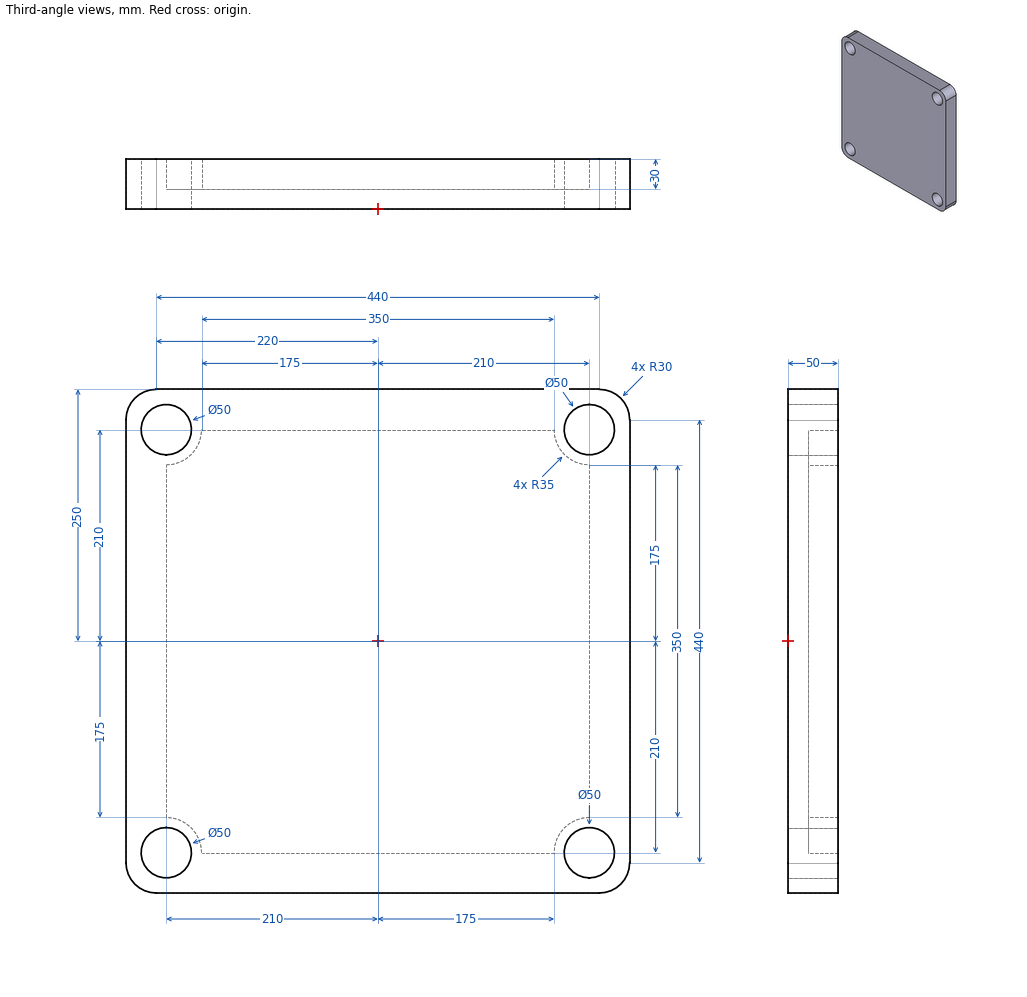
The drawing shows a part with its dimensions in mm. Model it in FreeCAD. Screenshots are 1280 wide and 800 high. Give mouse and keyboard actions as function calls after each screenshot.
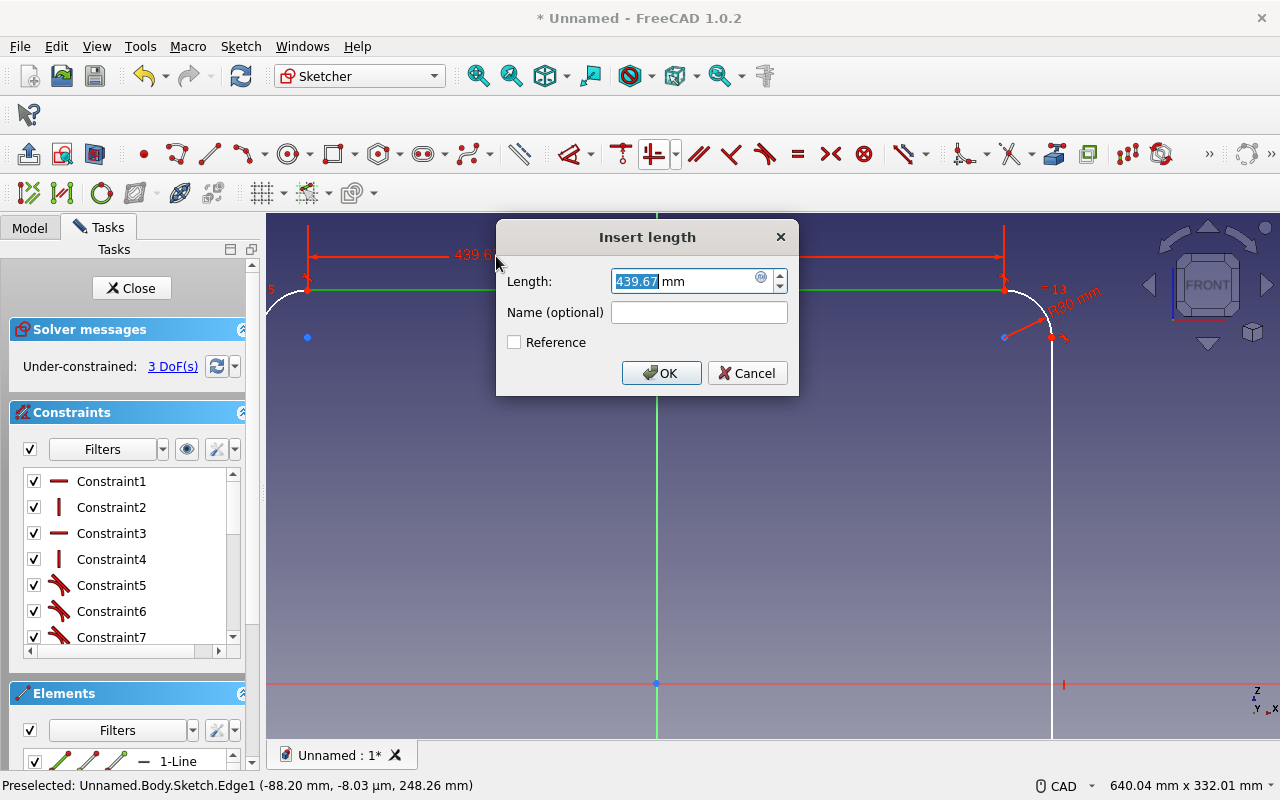
text(440)
key(Return)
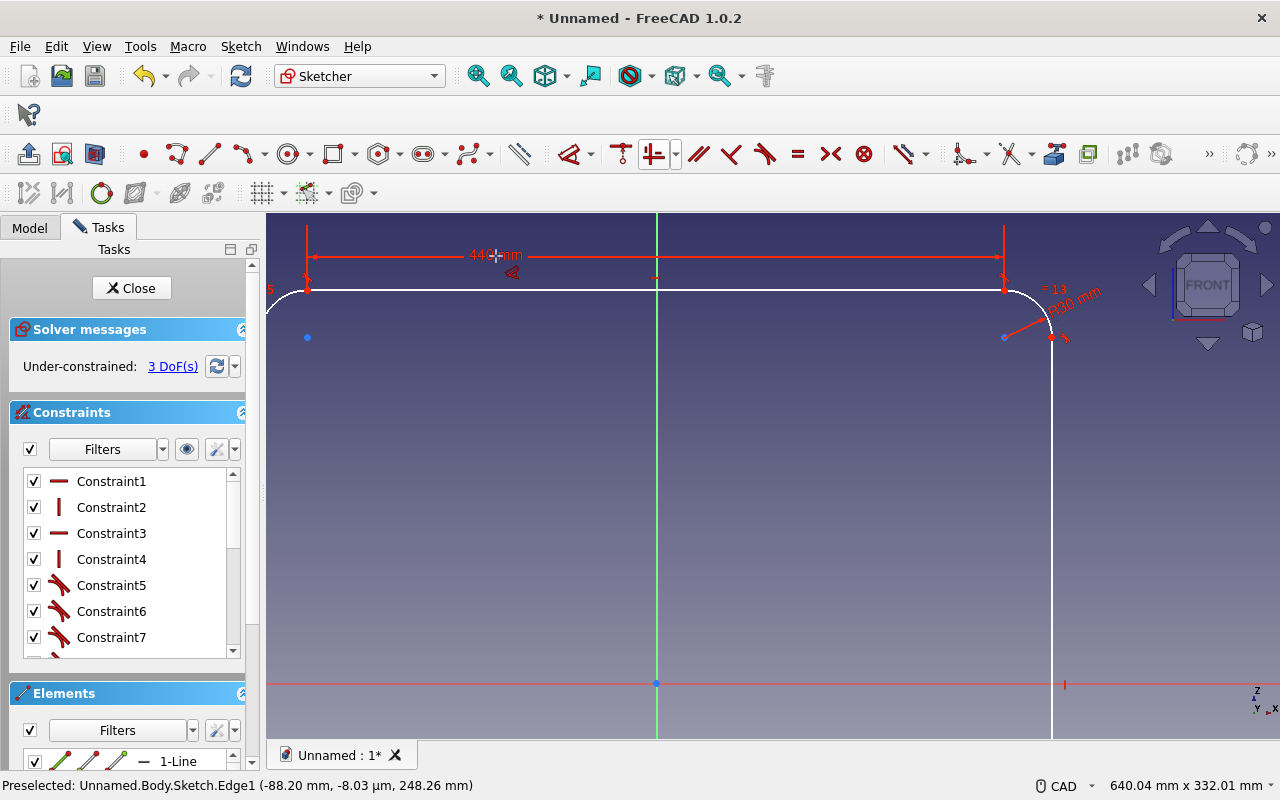
click(1052, 546)
click(1086, 524)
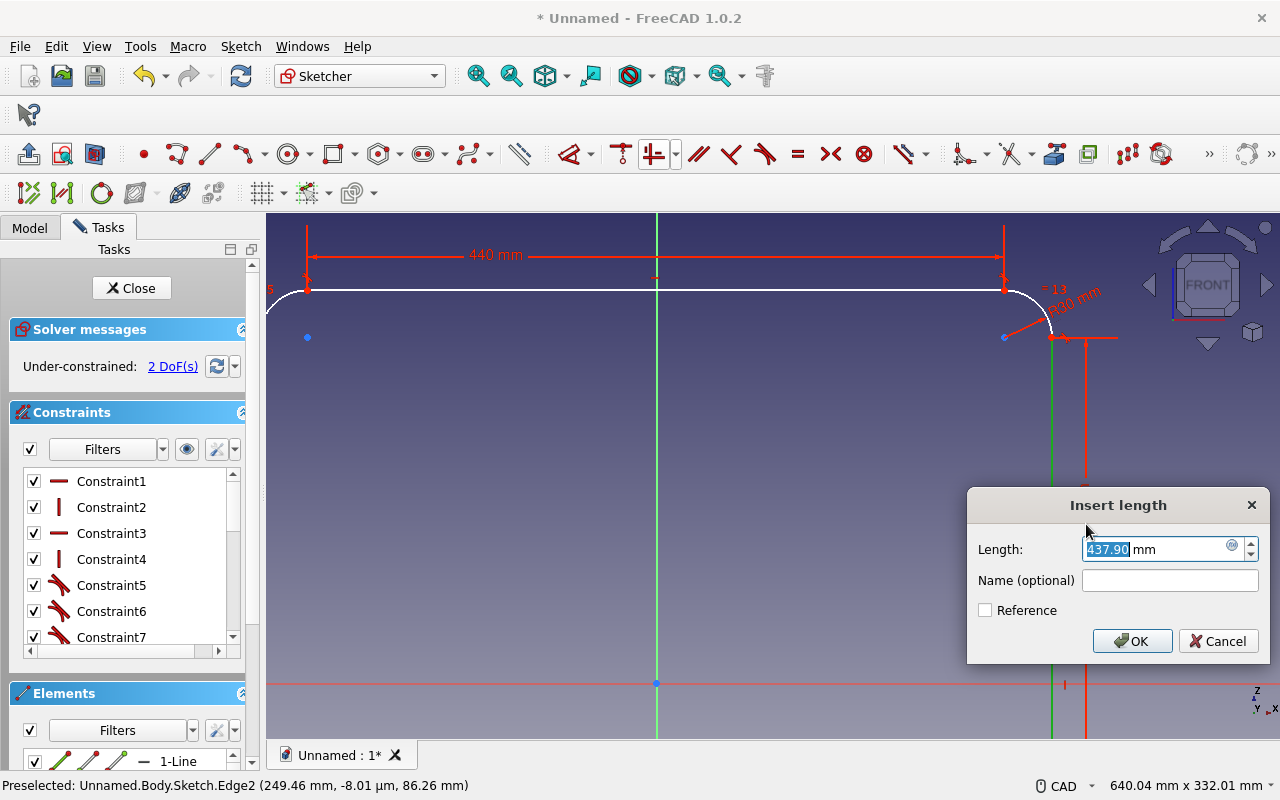
text(440)
key(Return)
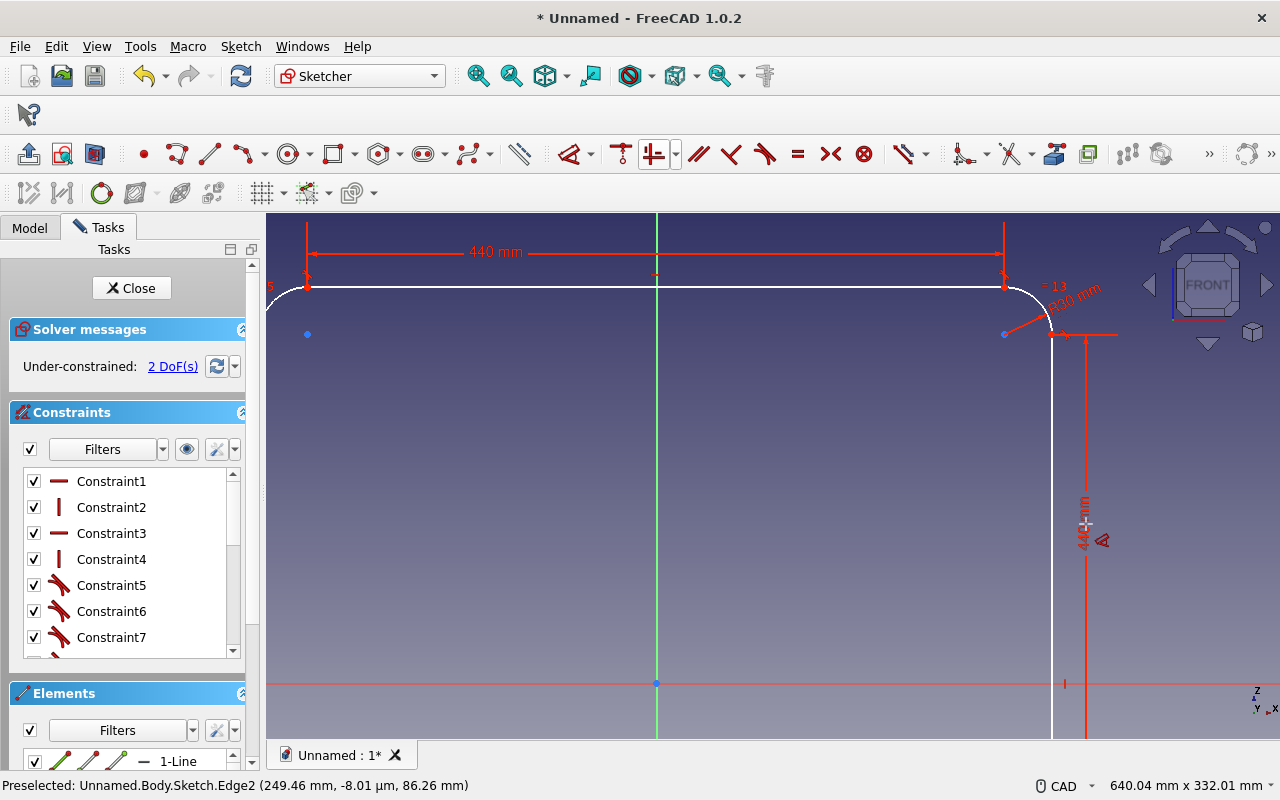
click(307, 287)
click(402, 253)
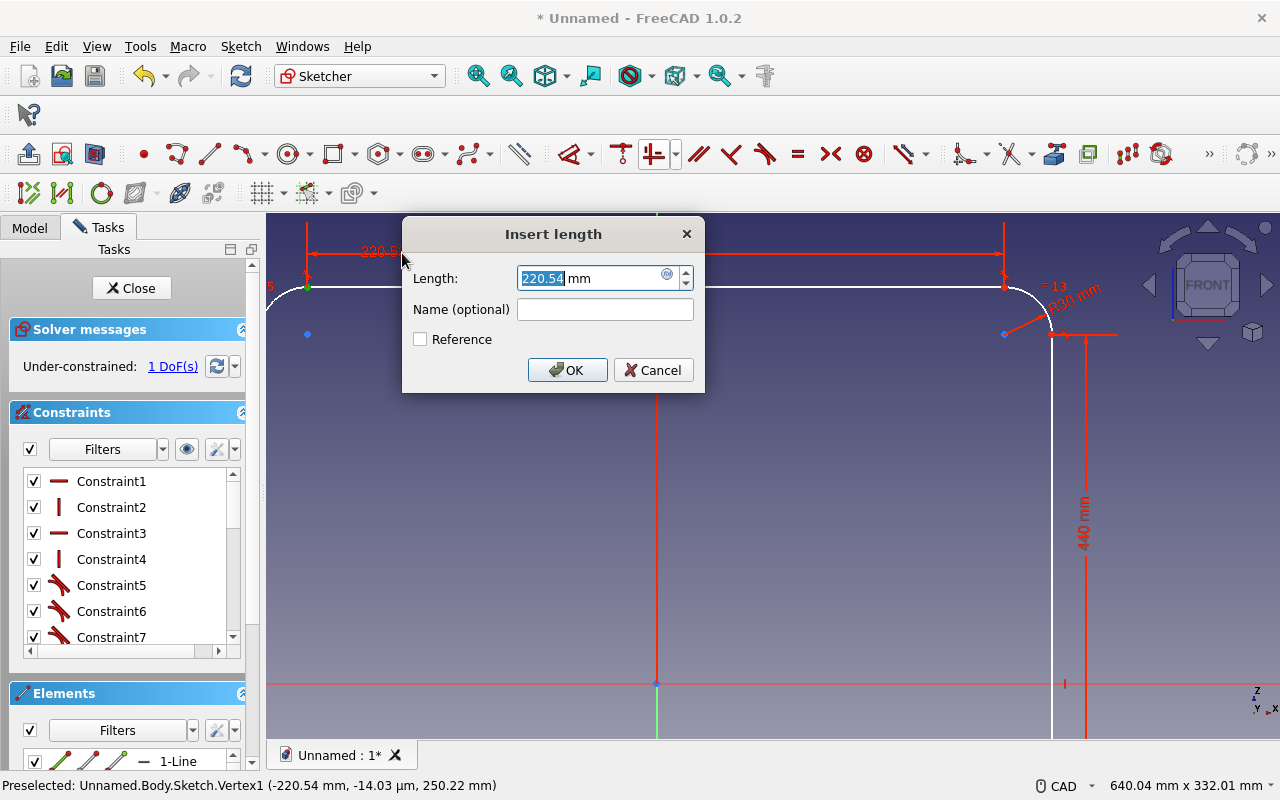
text(220)
key(Return)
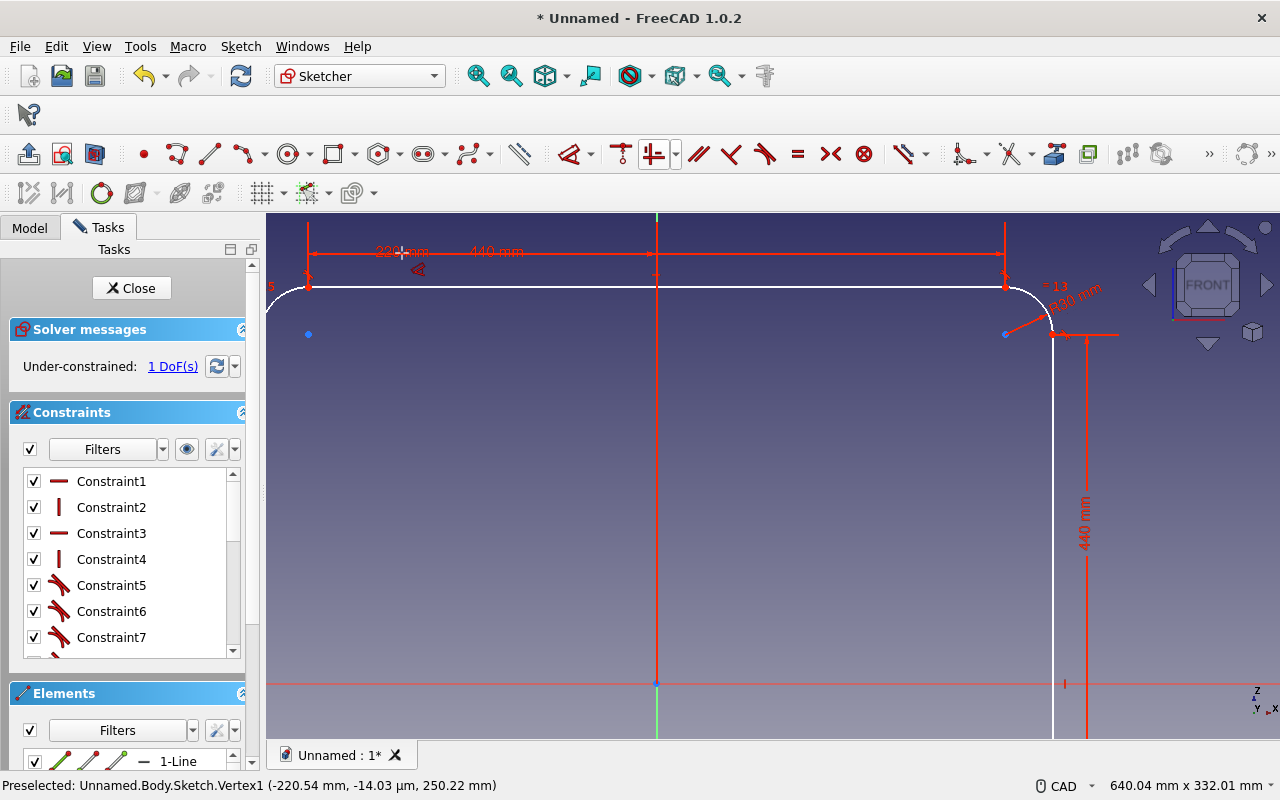
click(308, 287)
click(691, 485)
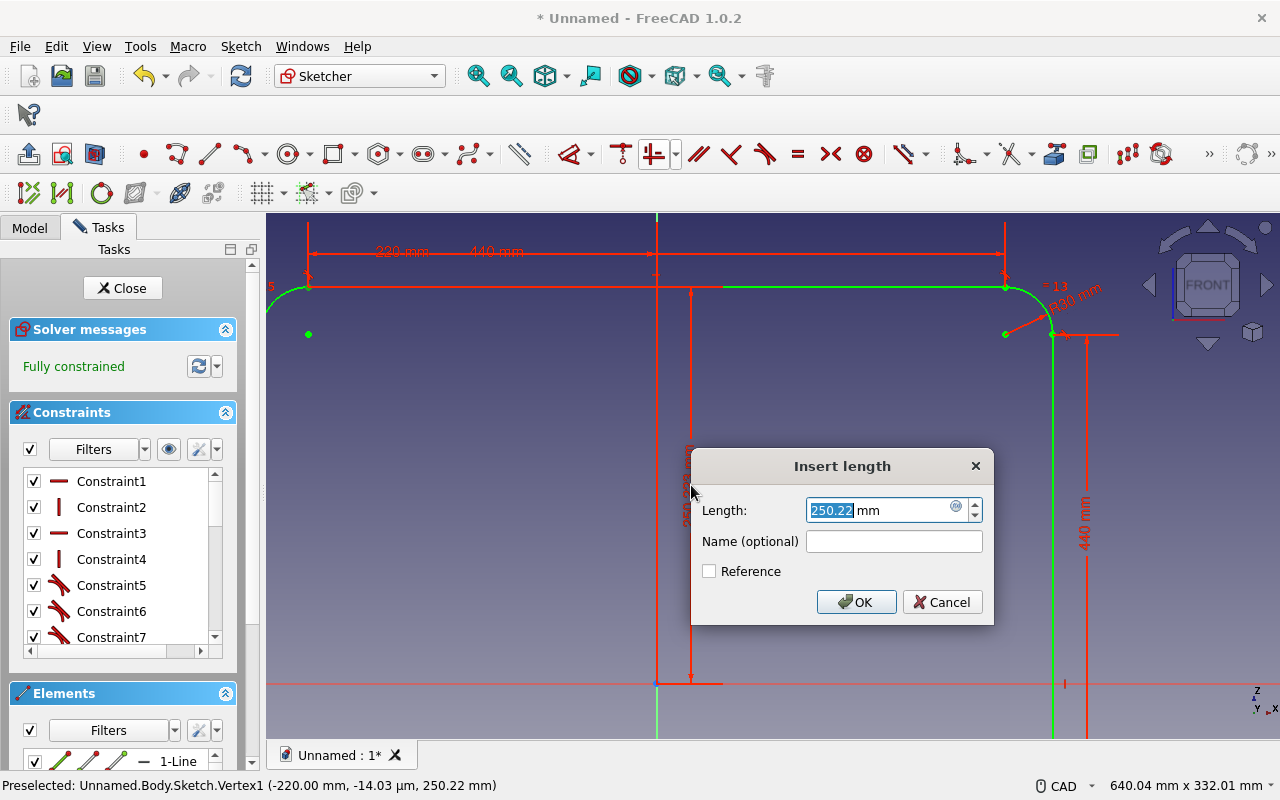
text(250)
key(Return)
key(Escape)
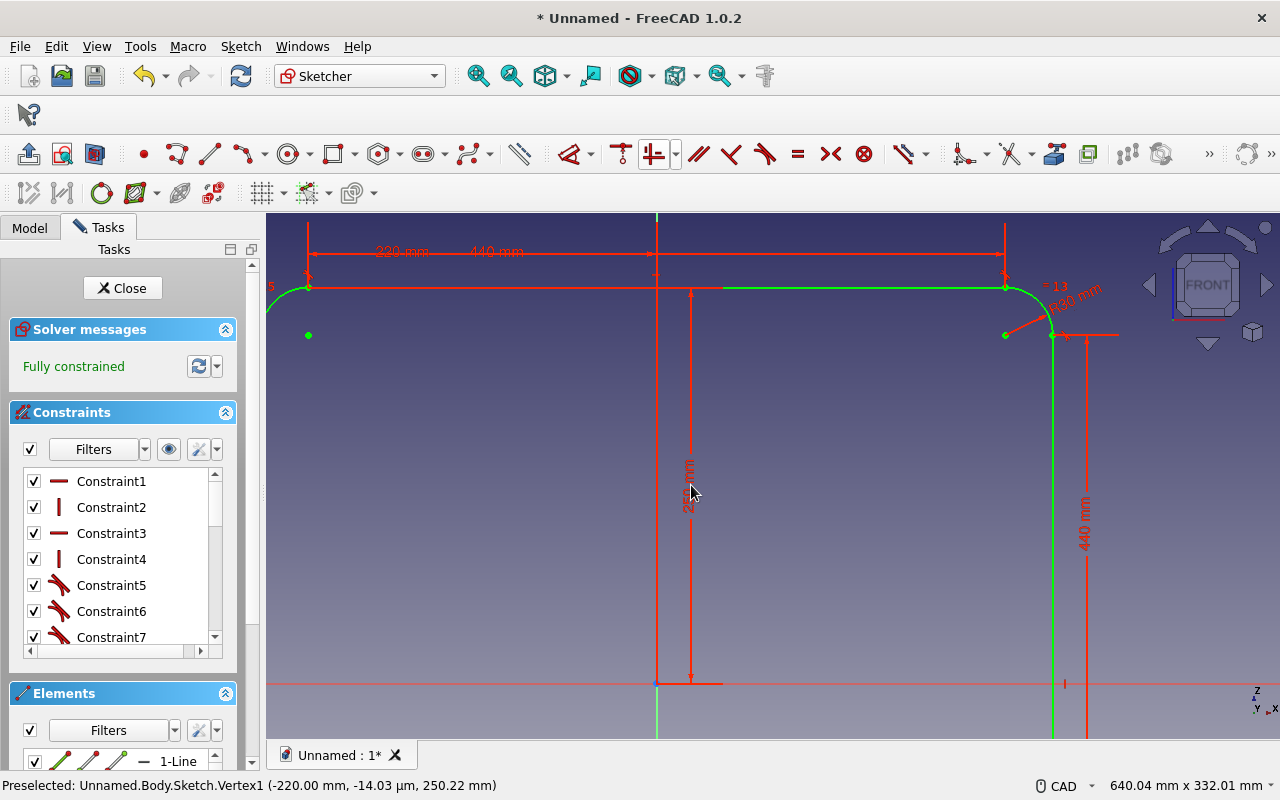
click(123, 288)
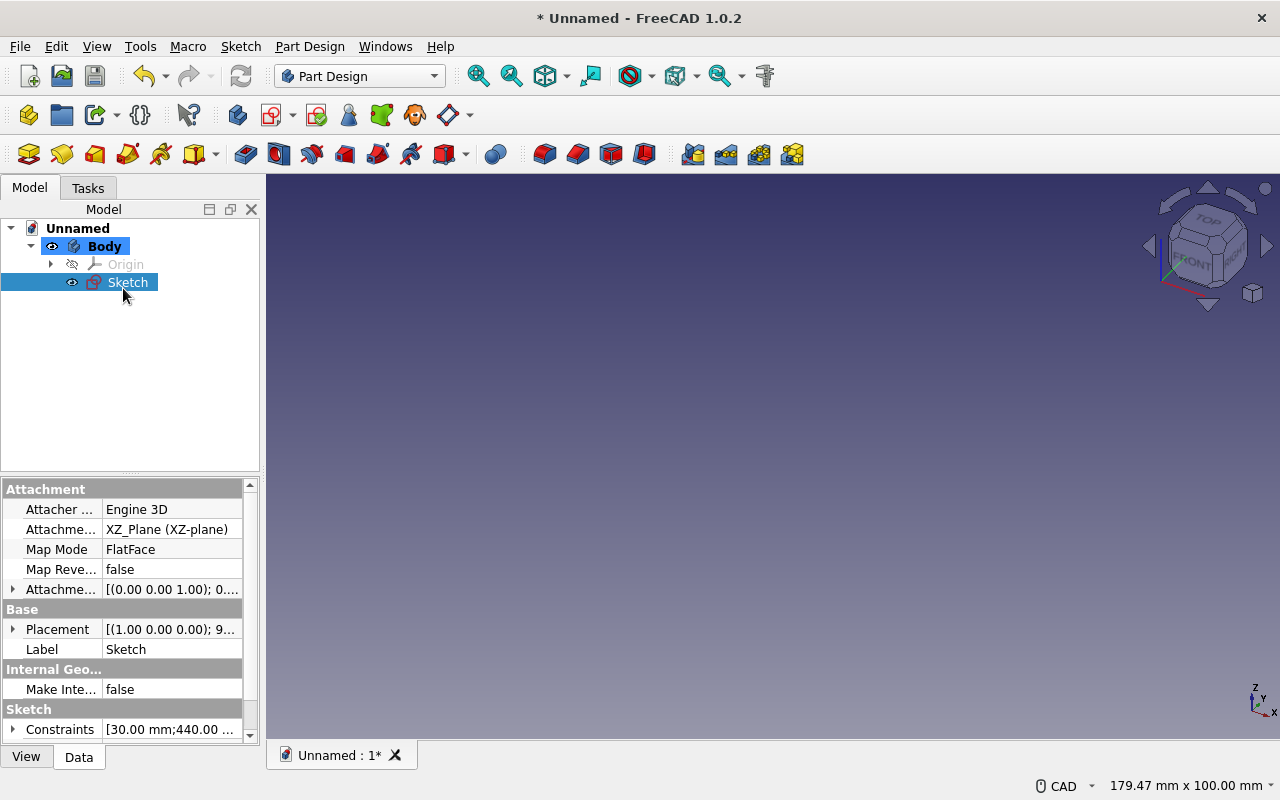
click(29, 154)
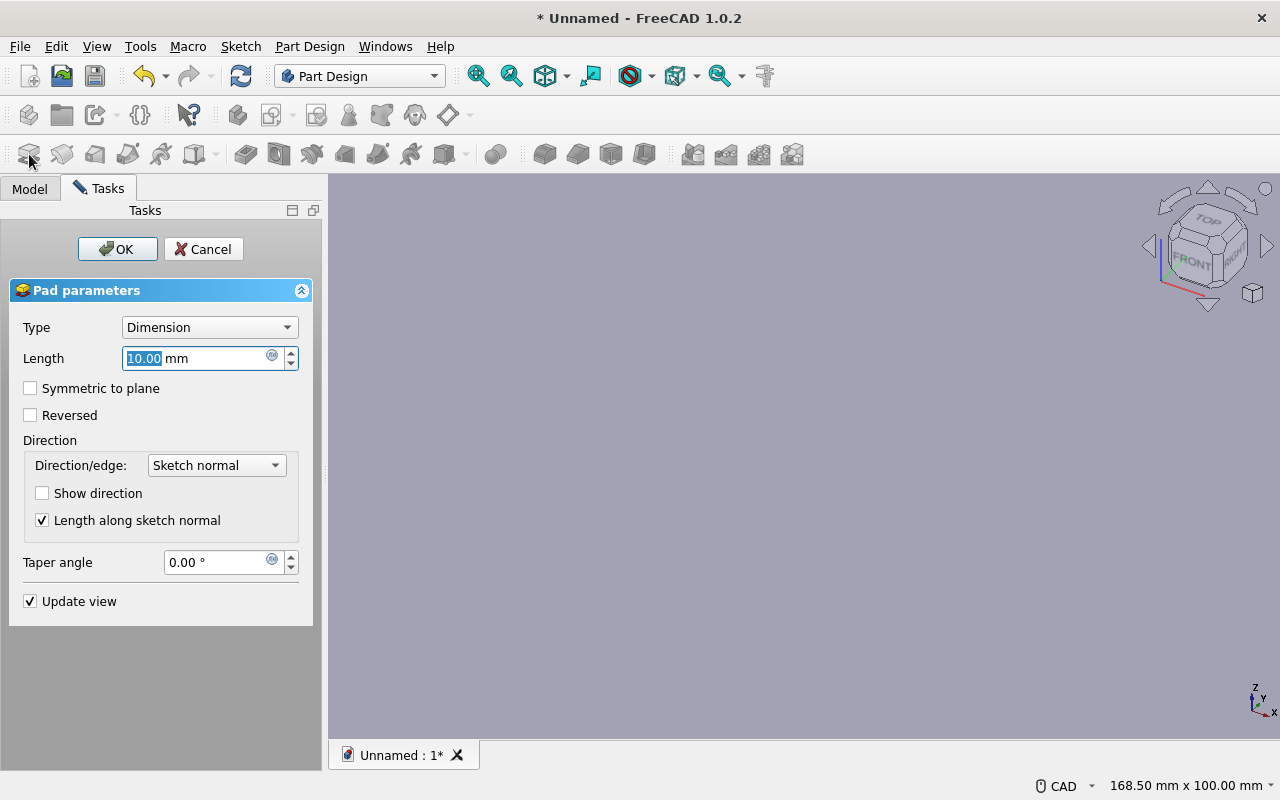
text(50)
key(Tab)